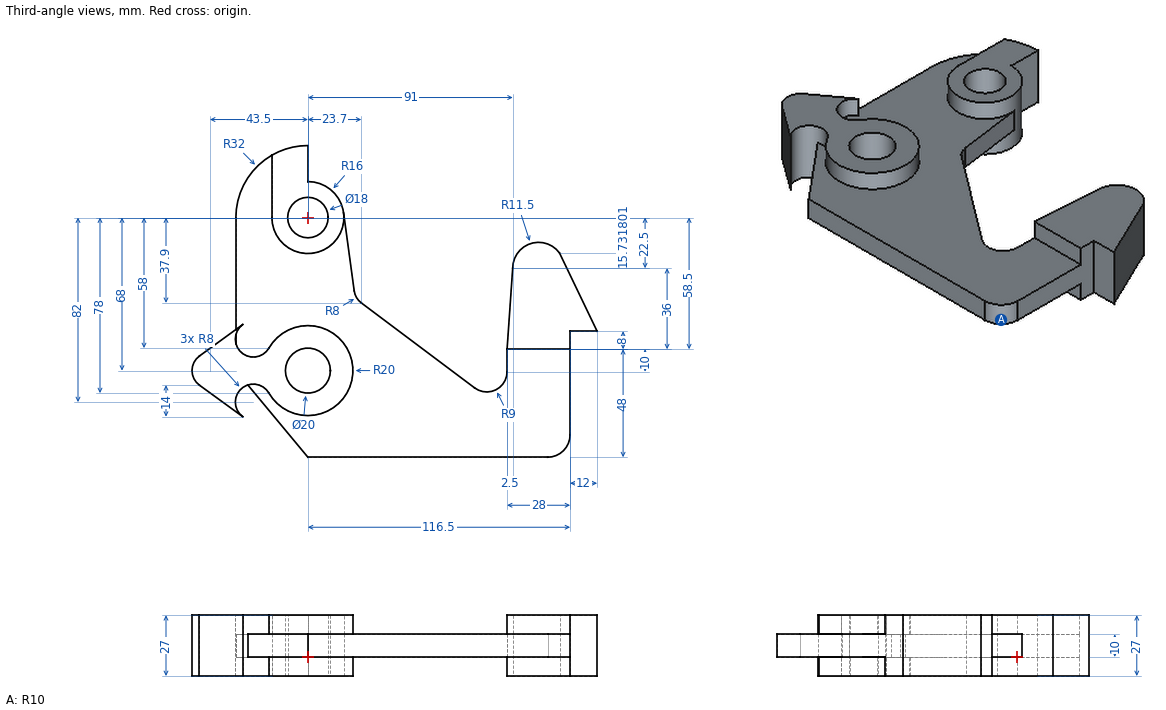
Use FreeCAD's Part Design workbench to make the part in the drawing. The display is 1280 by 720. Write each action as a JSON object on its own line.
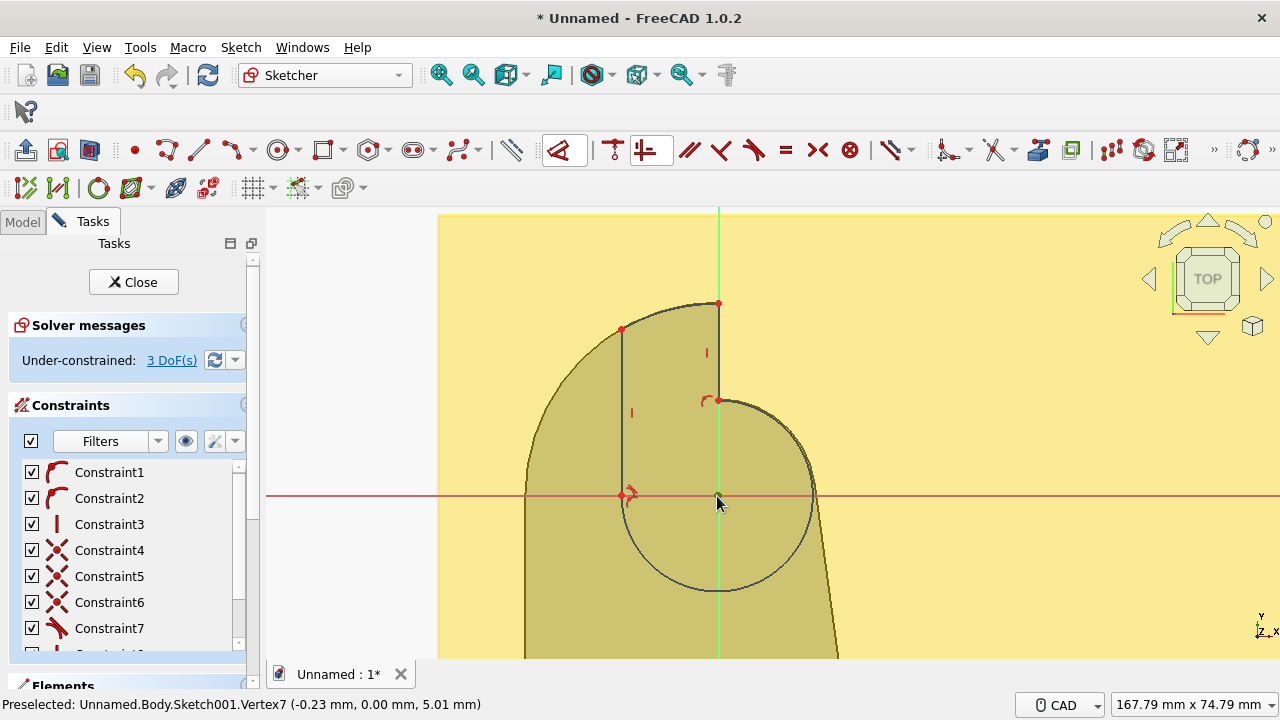
{"action": "left_click", "coordinate": [719, 546]}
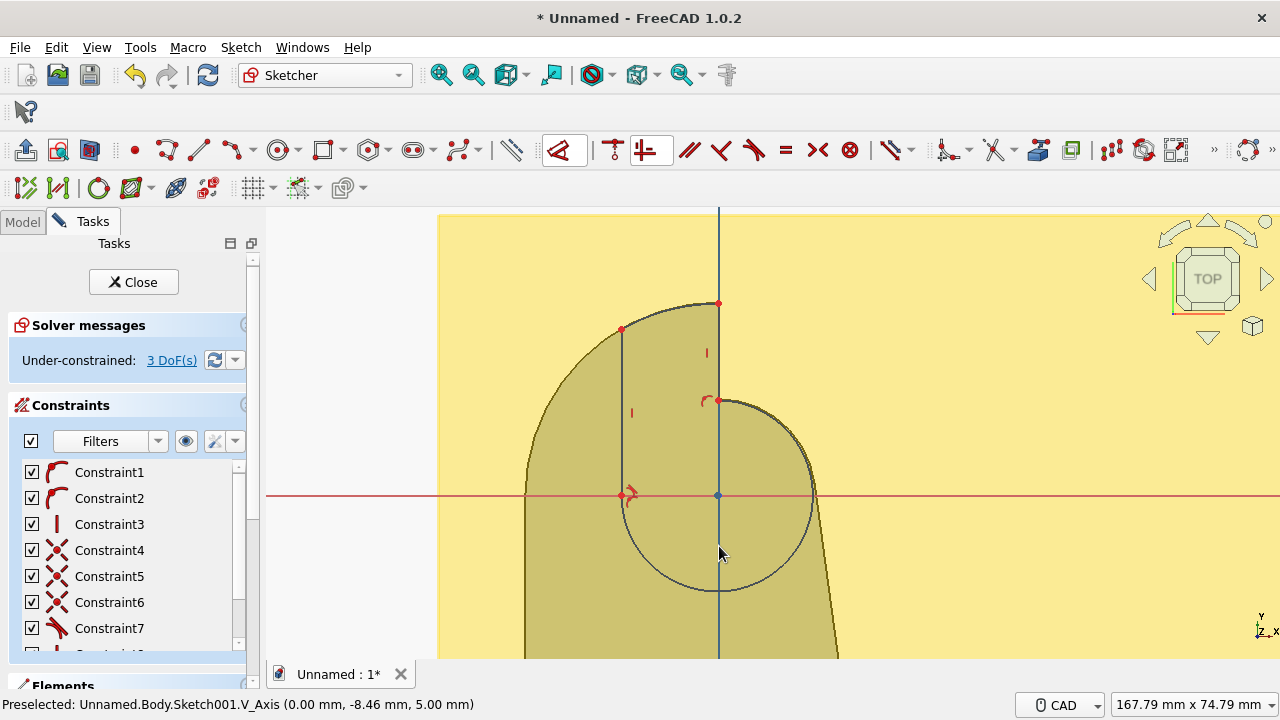
{"action": "left_click", "coordinate": [614, 150]}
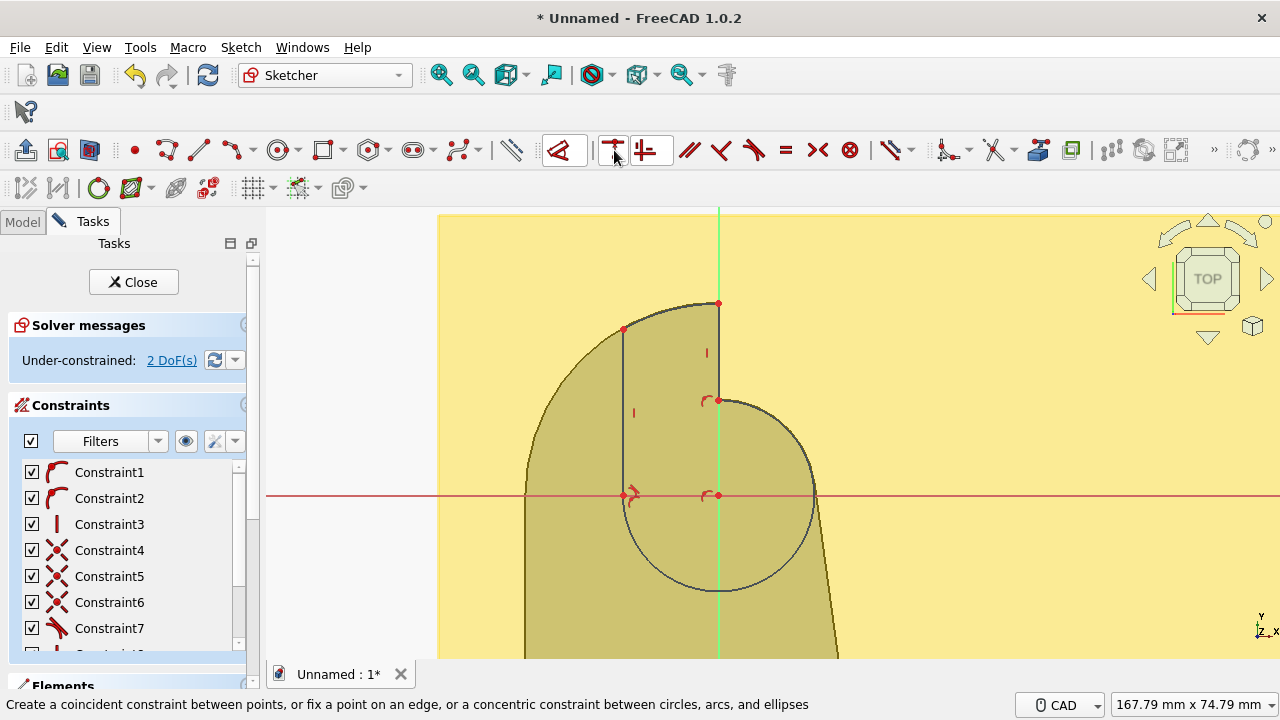
{"action": "left_click", "coordinate": [689, 306]}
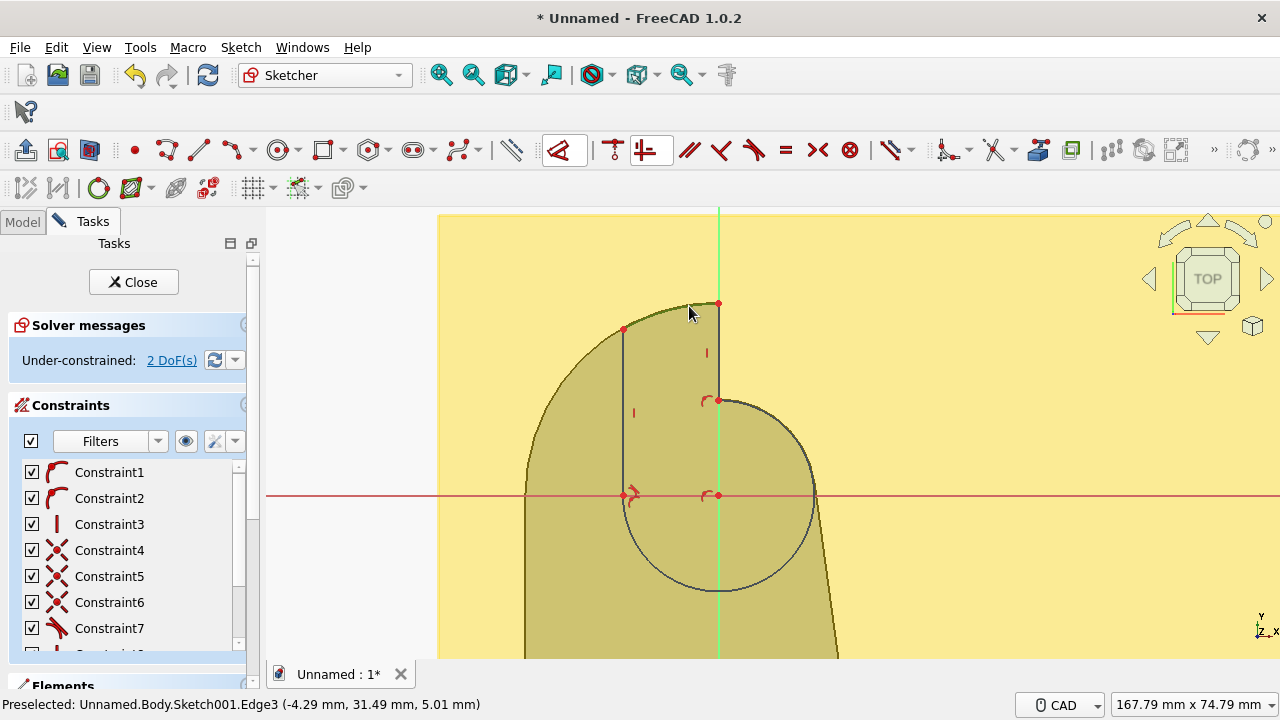
{"action": "left_click", "coordinate": [582, 150]}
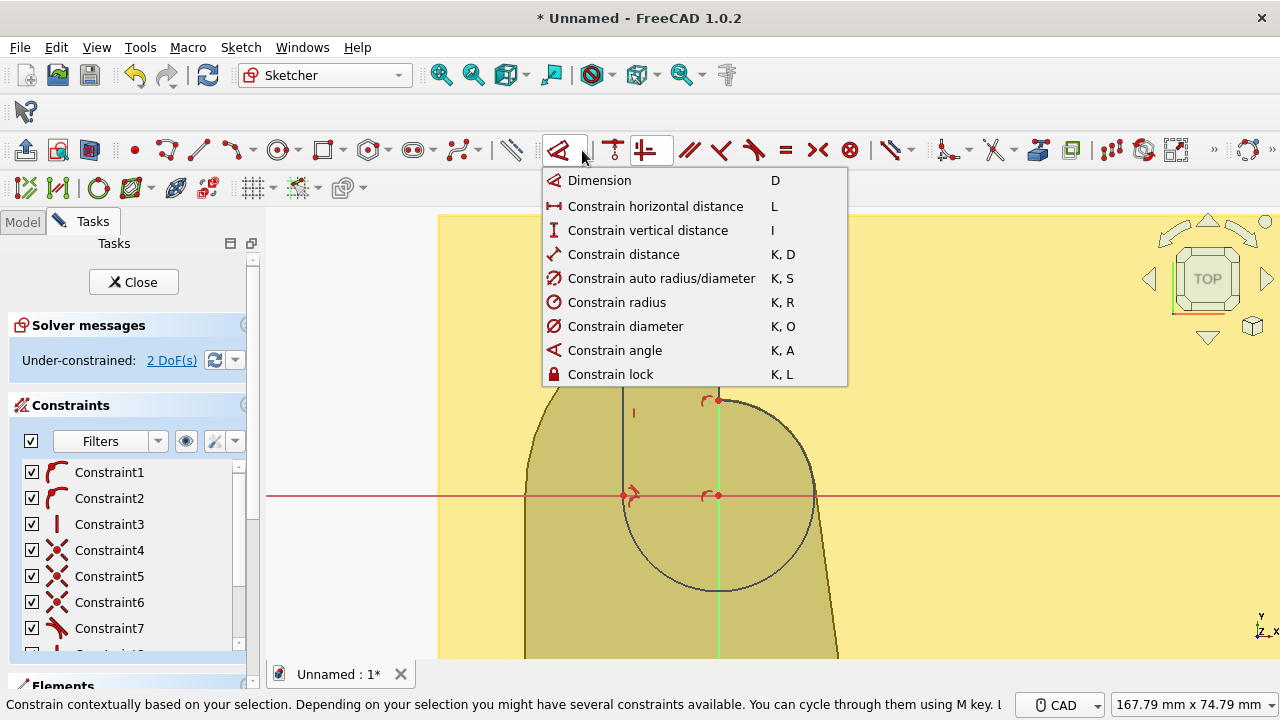
{"action": "left_click", "coordinate": [695, 302]}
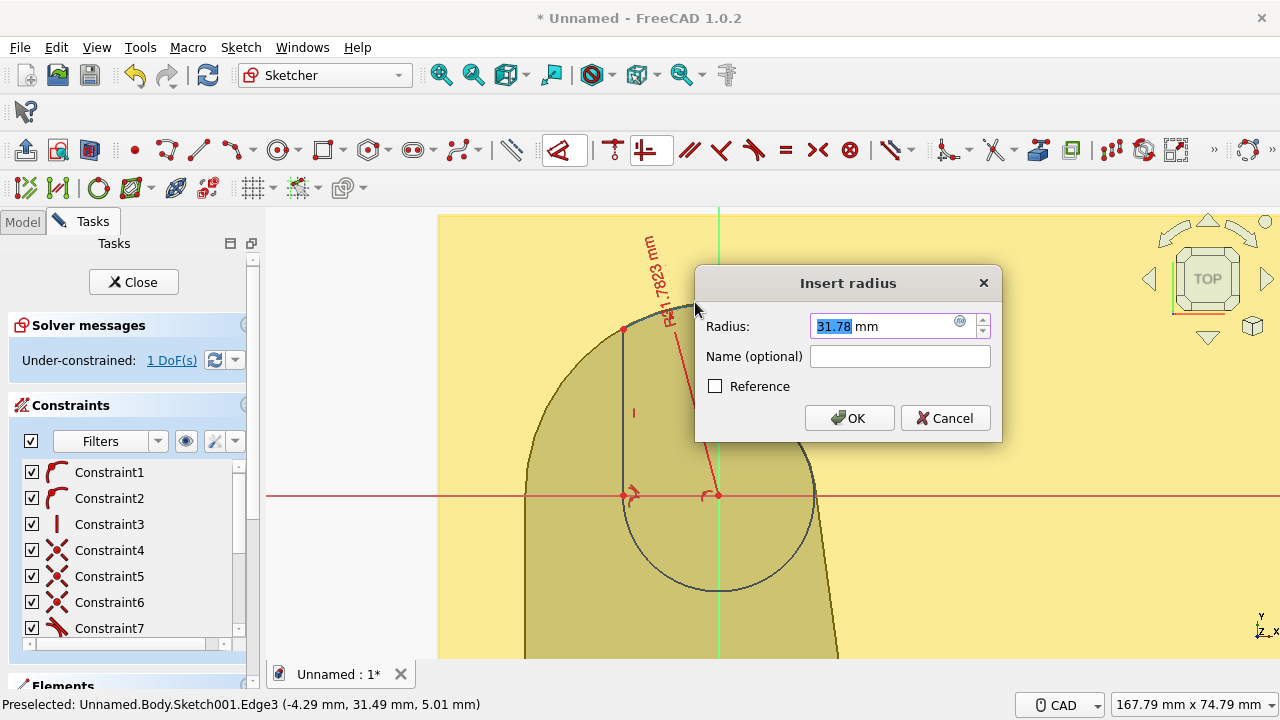
{"action": "type", "text": "32"}
{"action": "key", "text": "Return"}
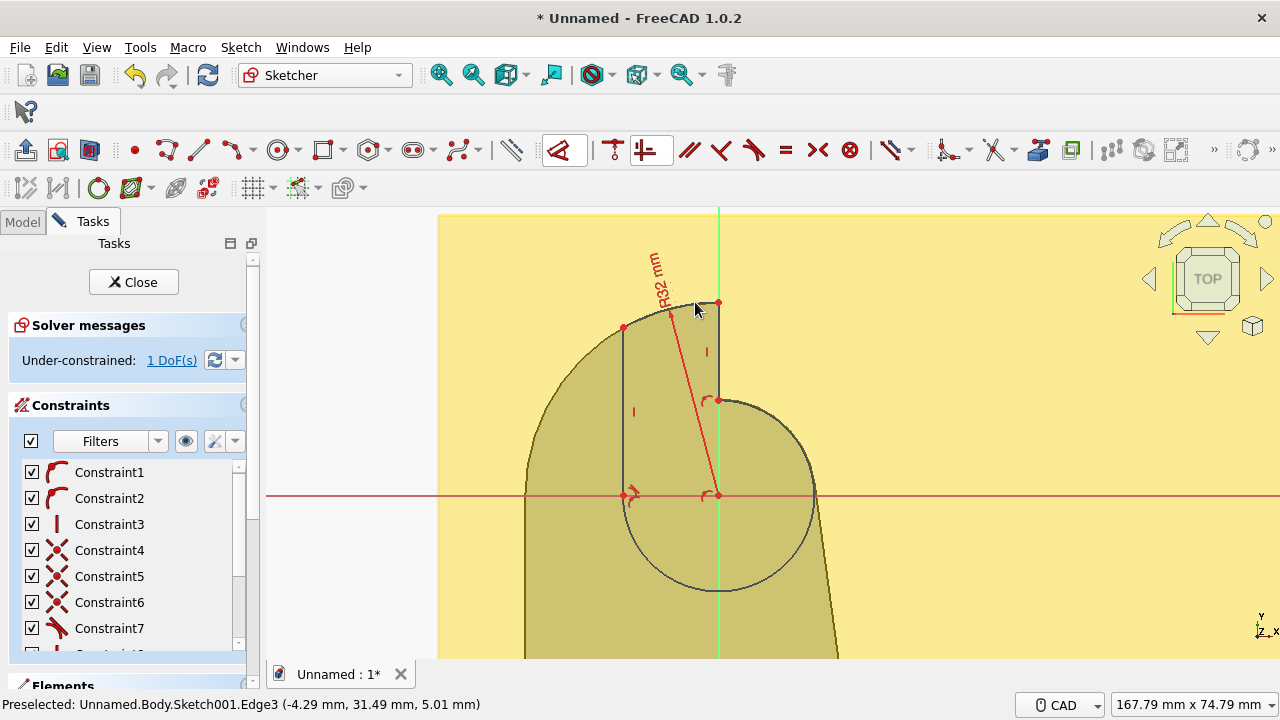
{"action": "left_click", "coordinate": [704, 590]}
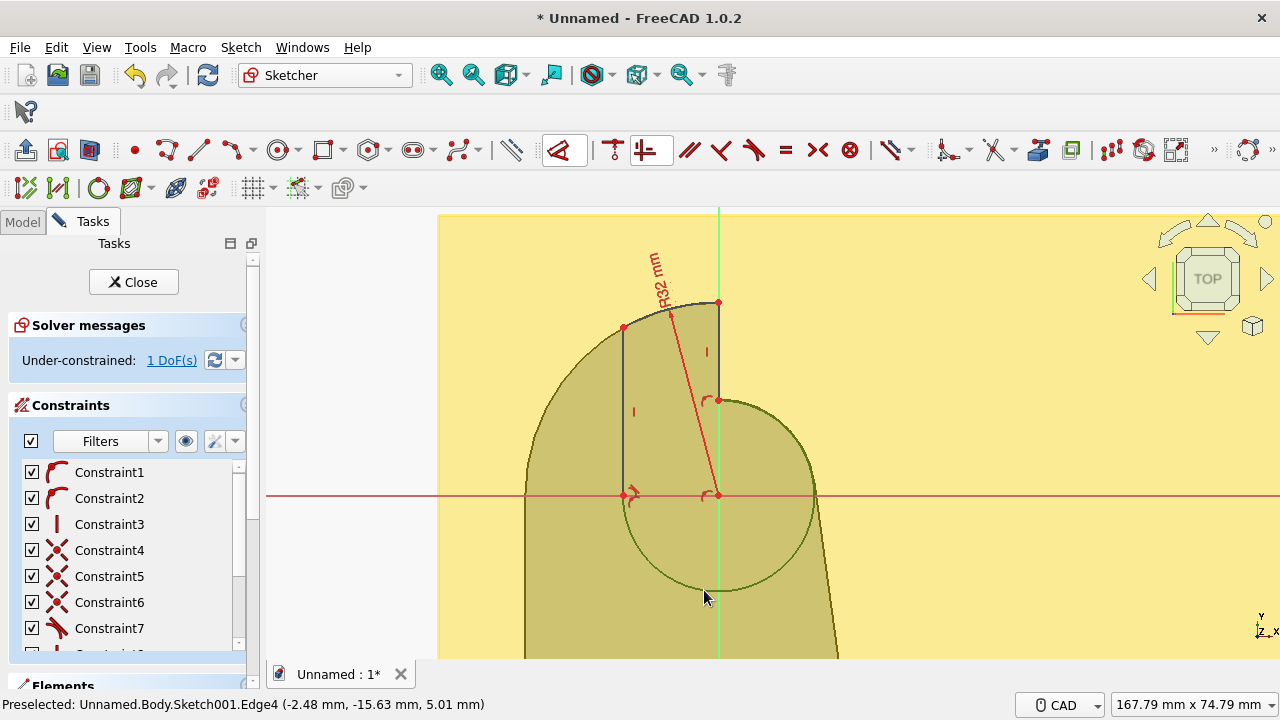
{"action": "key", "text": "k r"}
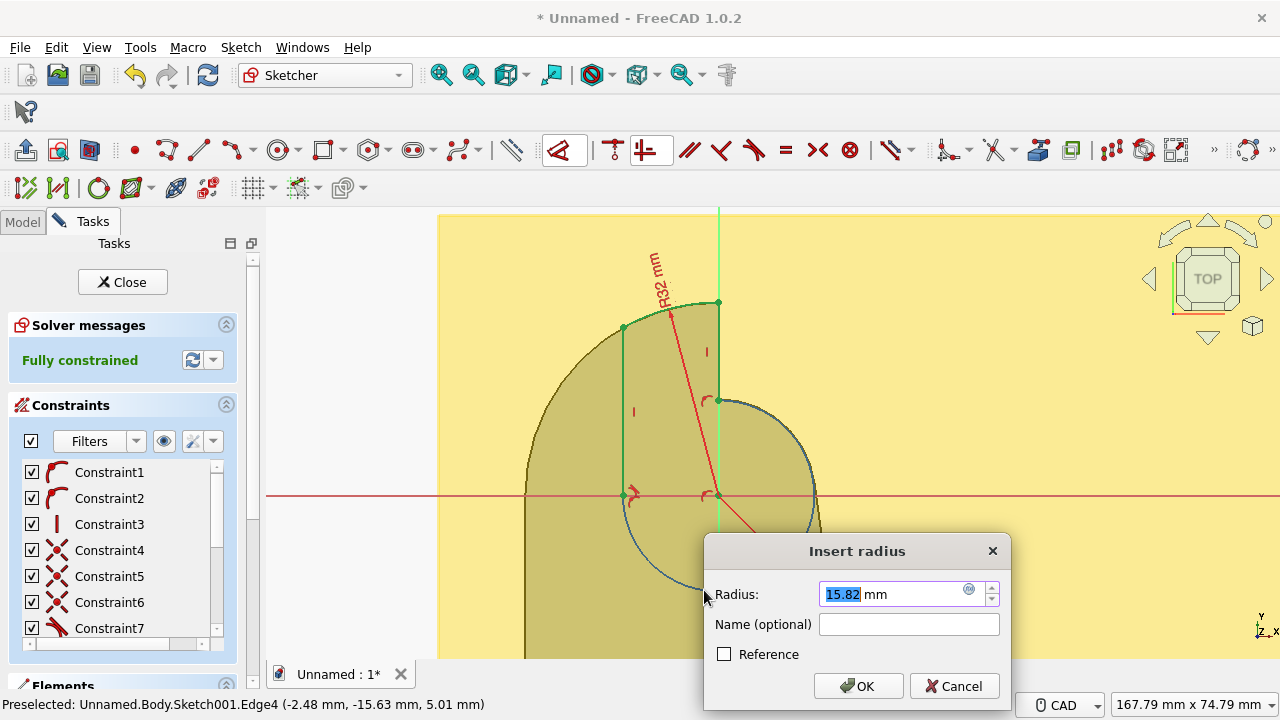
{"action": "type", "text": "16"}
{"action": "key", "text": "Return"}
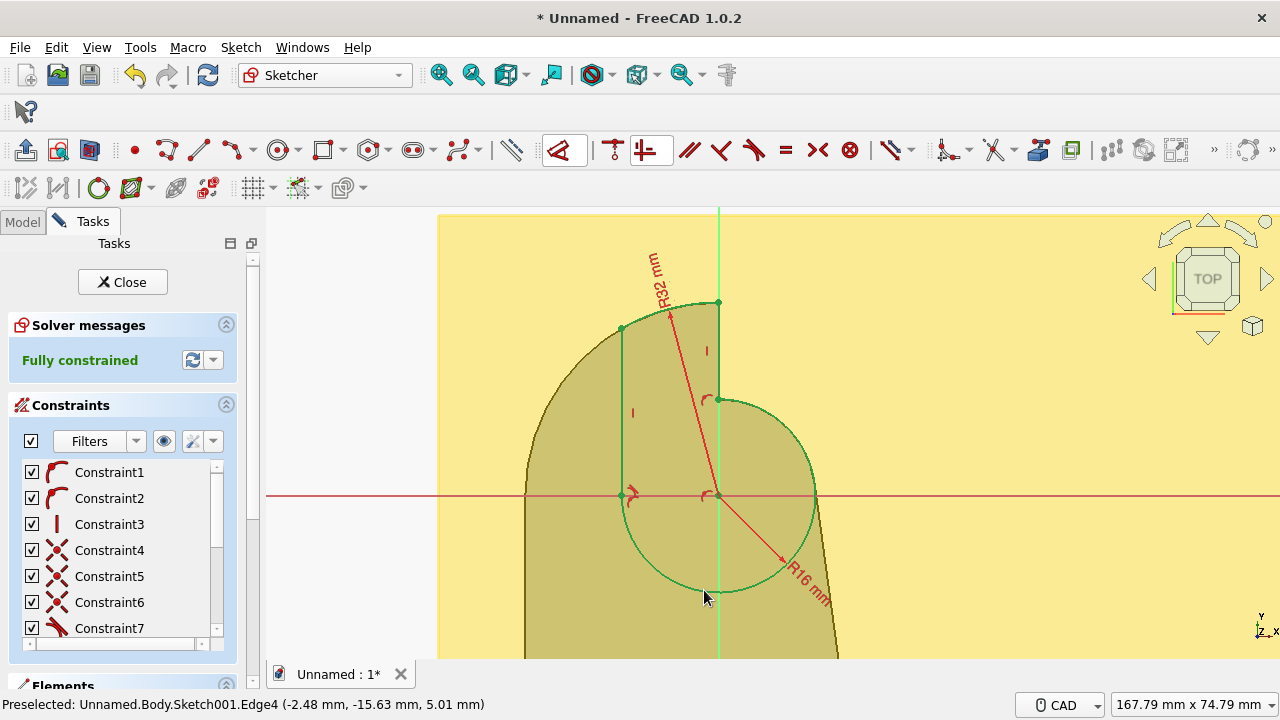
{"action": "left_click", "coordinate": [123, 282]}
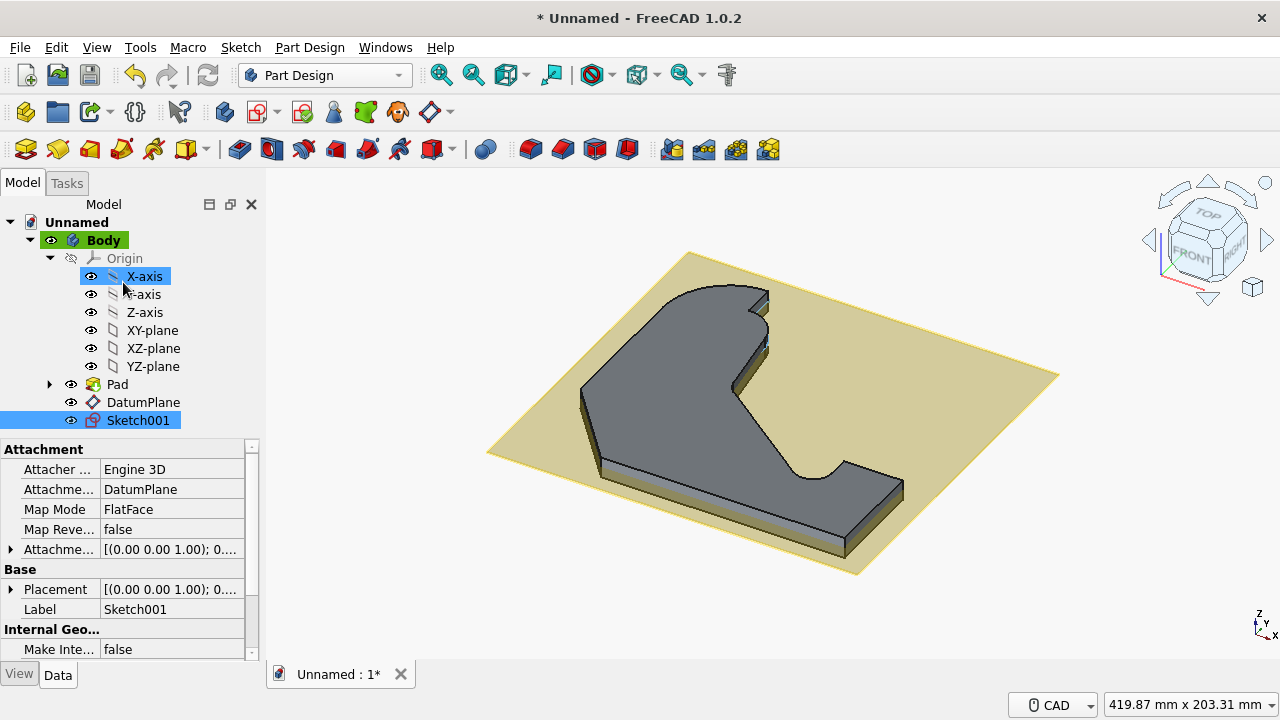
{"action": "left_click", "coordinate": [26, 150]}